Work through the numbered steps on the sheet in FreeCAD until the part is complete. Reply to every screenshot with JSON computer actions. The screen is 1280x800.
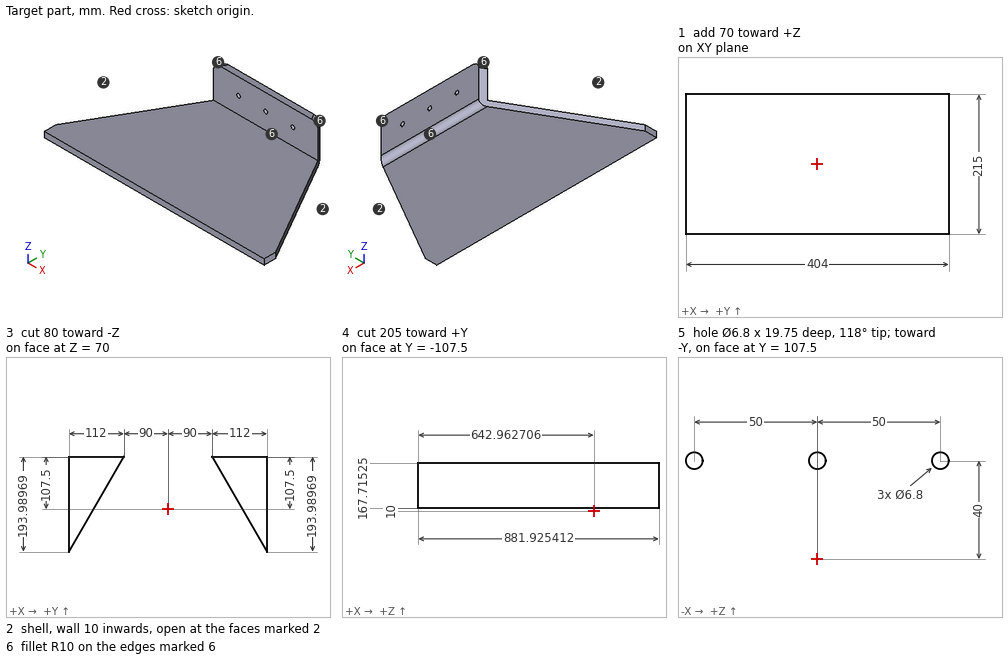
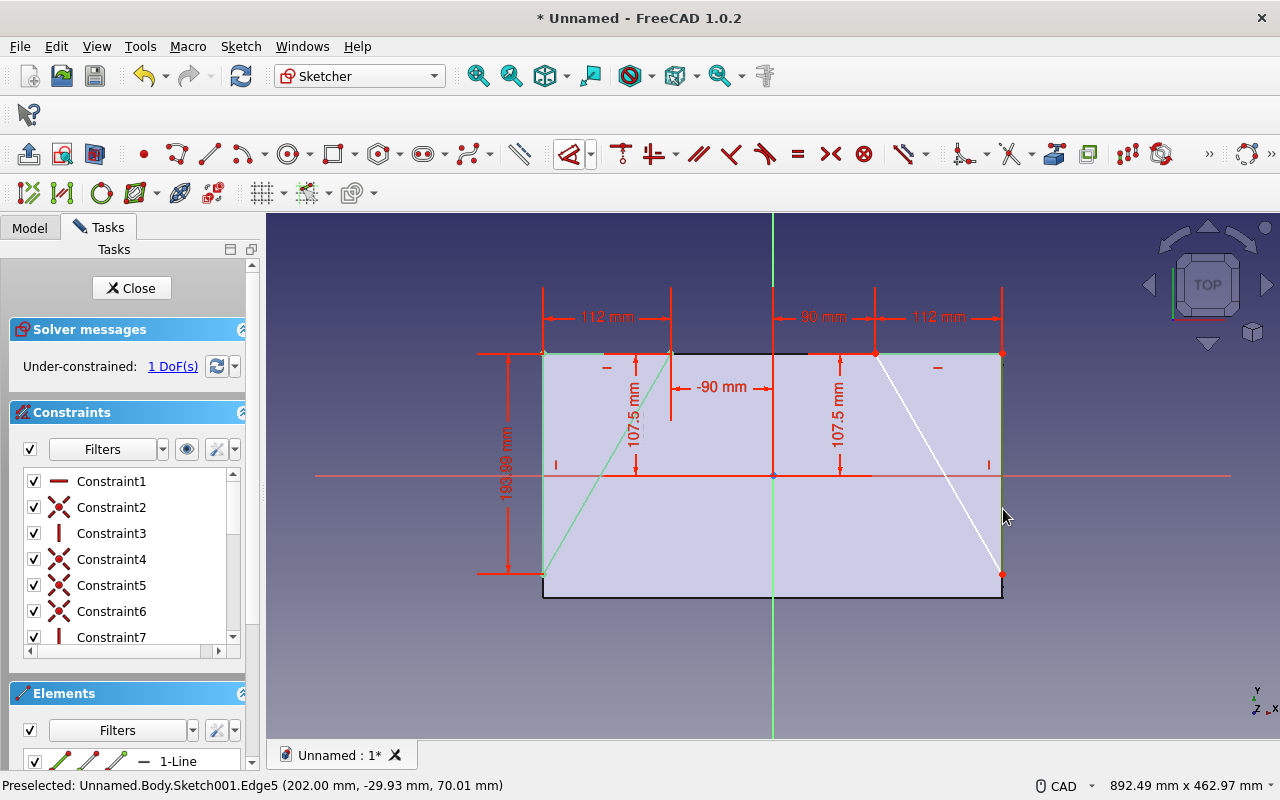
{"action": "left_click", "coordinate": [590, 154]}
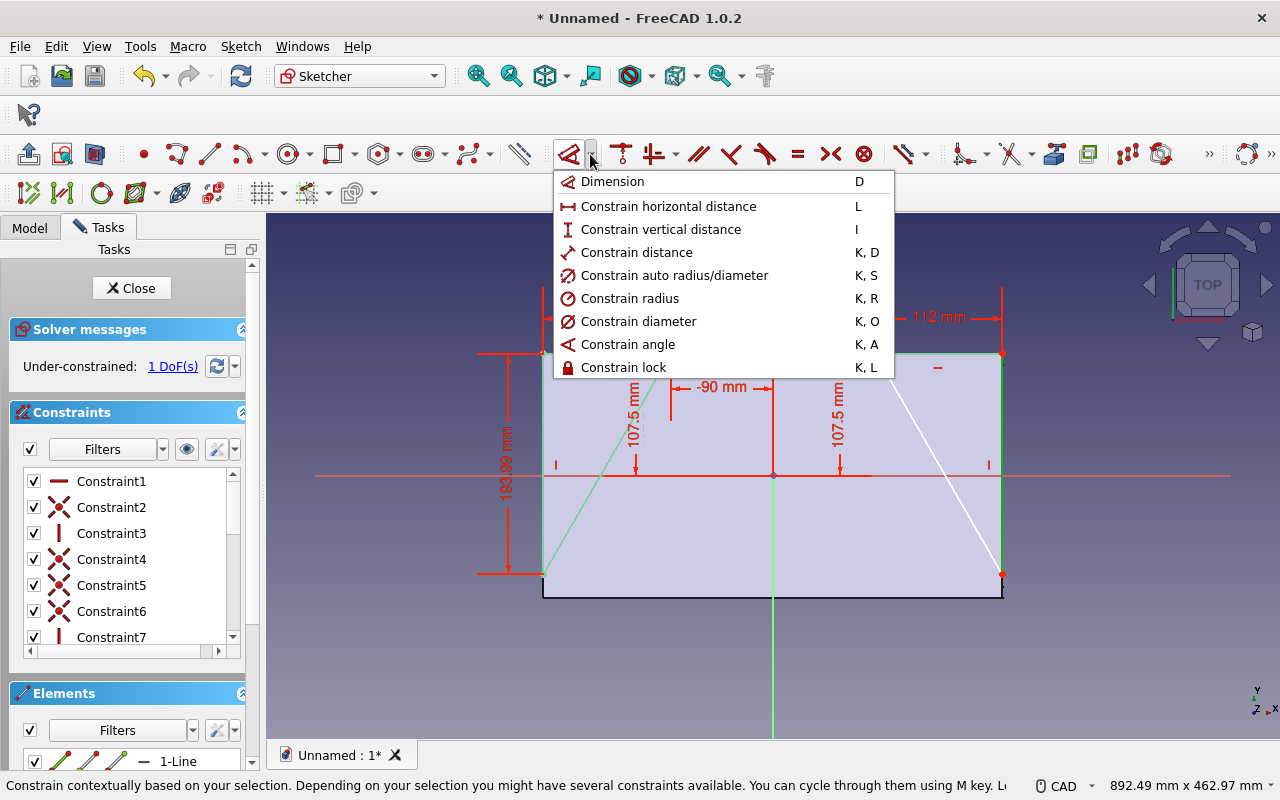
{"action": "left_click", "coordinate": [724, 230]}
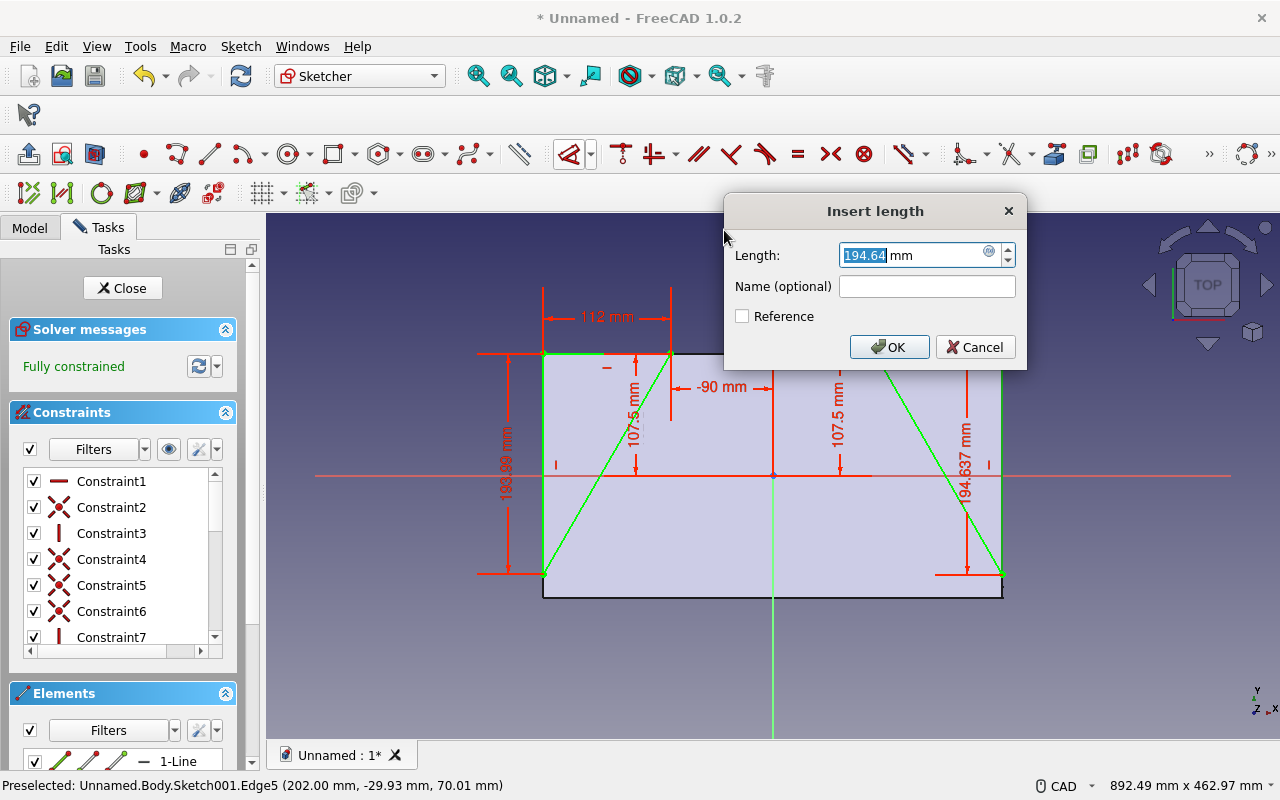
{"action": "type", "text": "193.98969"}
{"action": "key", "text": "Return"}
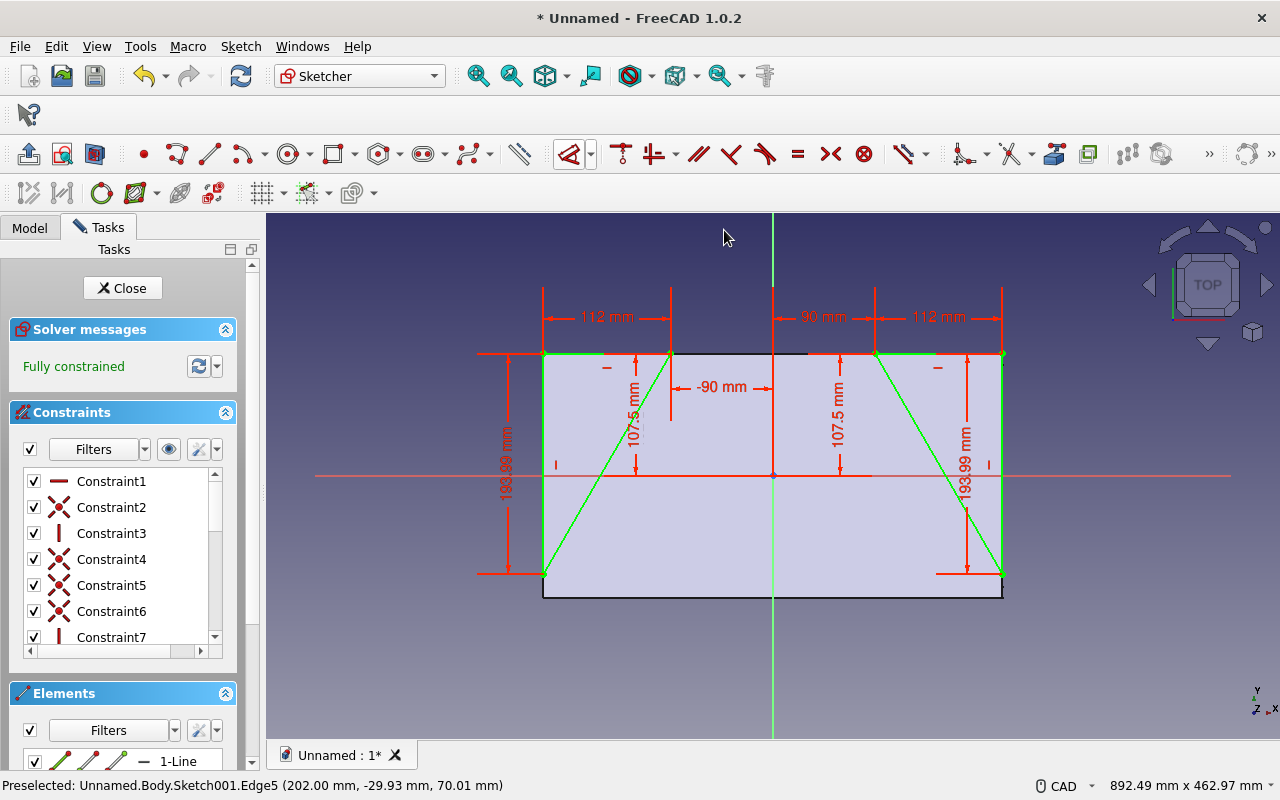
{"action": "left_click", "coordinate": [123, 288]}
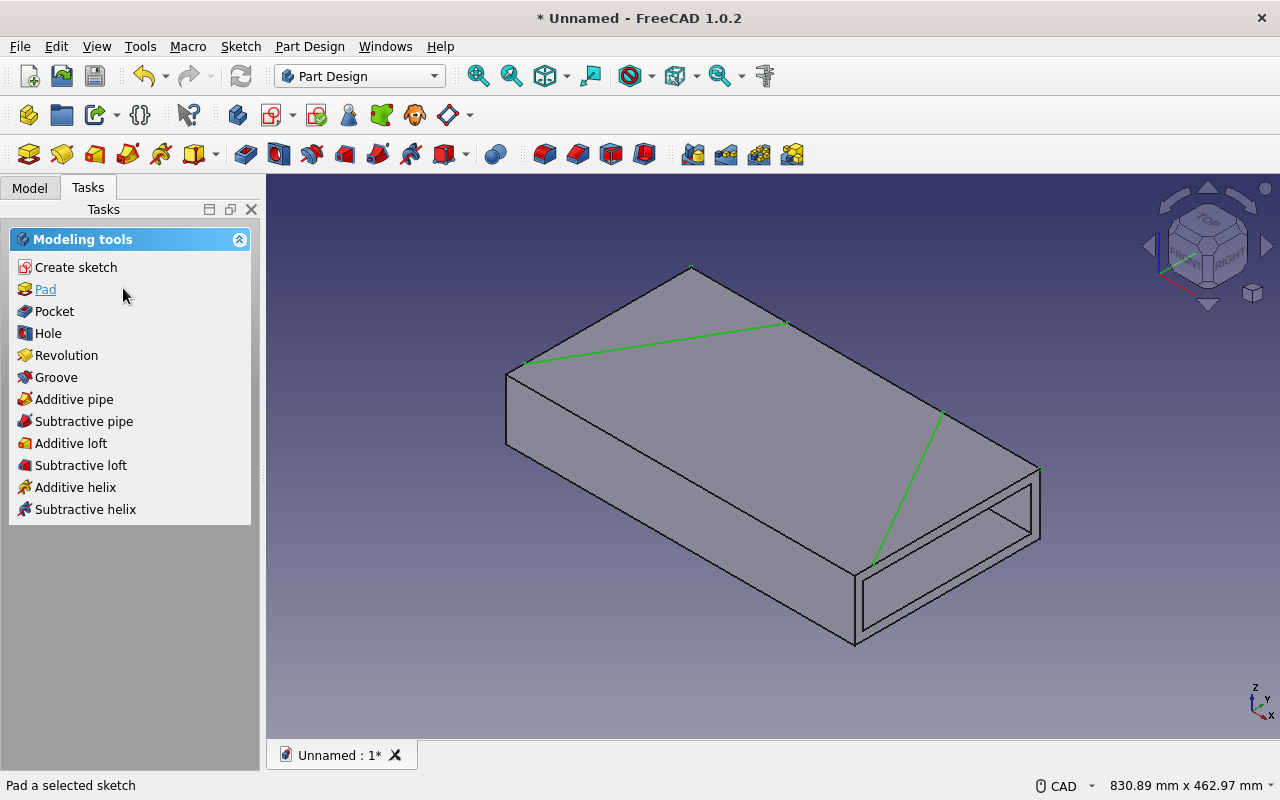
{"action": "left_click", "coordinate": [246, 154]}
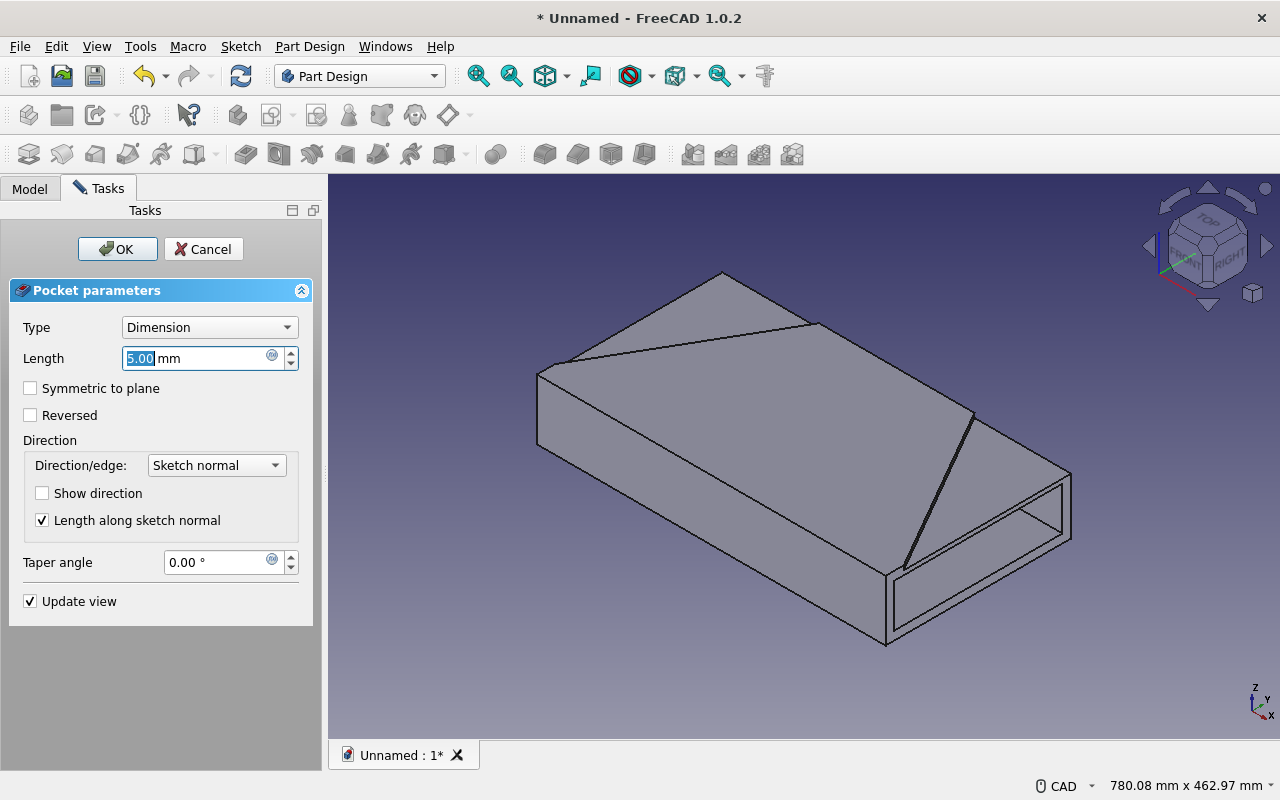
{"action": "type", "text": "80"}
{"action": "key", "text": "Tab"}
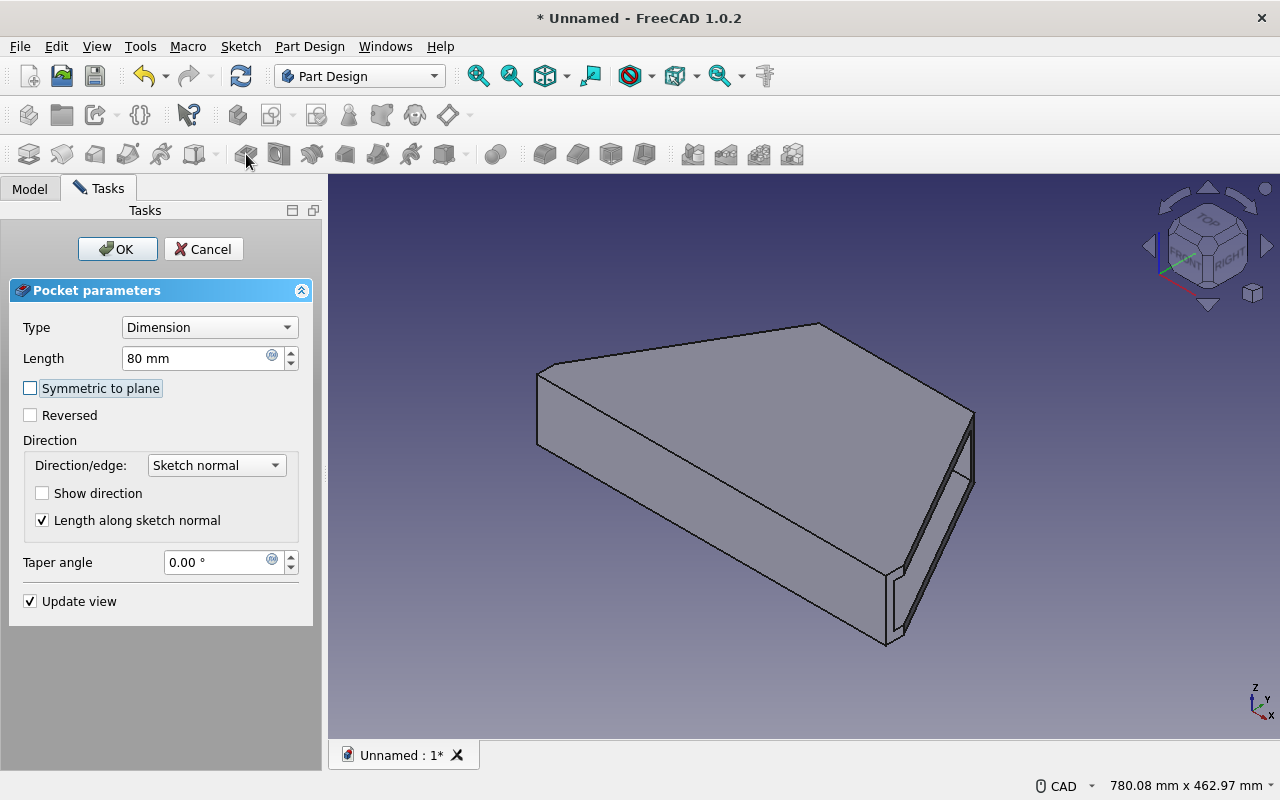
{"action": "left_click", "coordinate": [118, 249]}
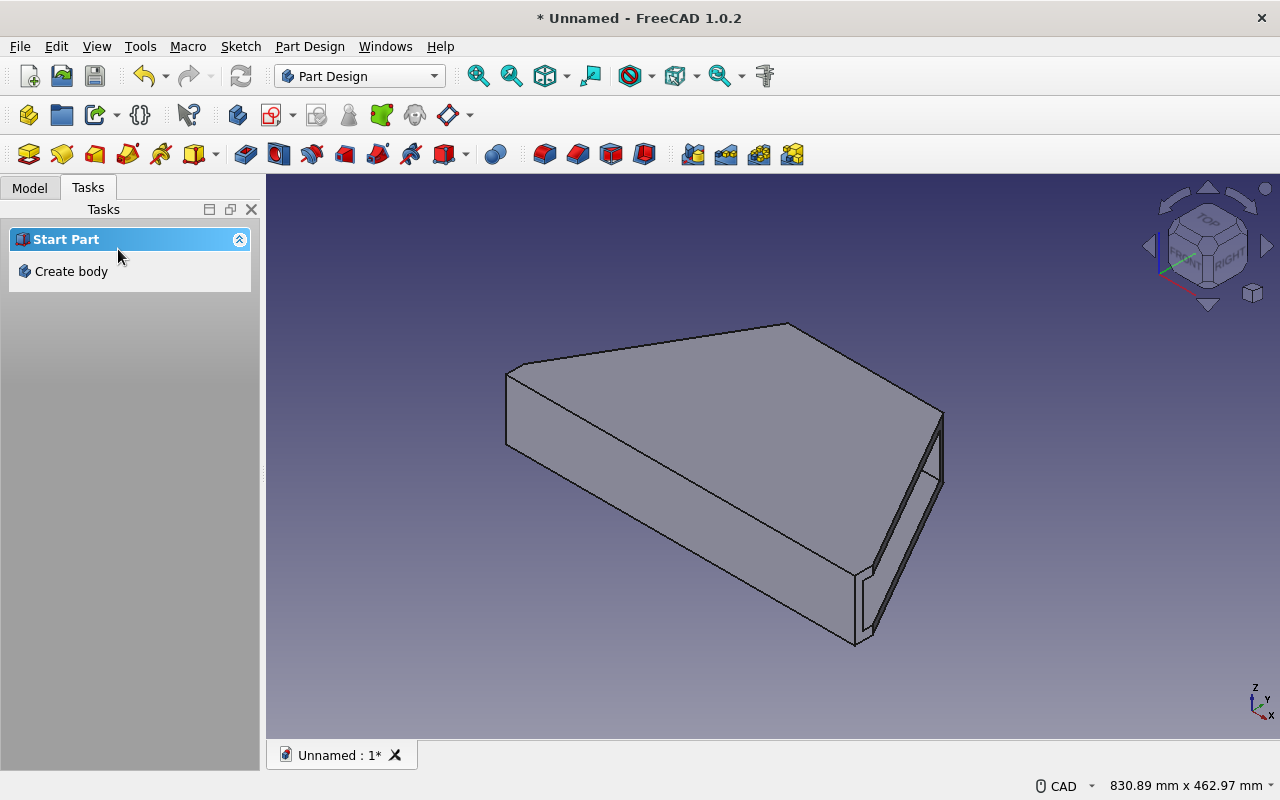
{"action": "left_click", "coordinate": [780, 567]}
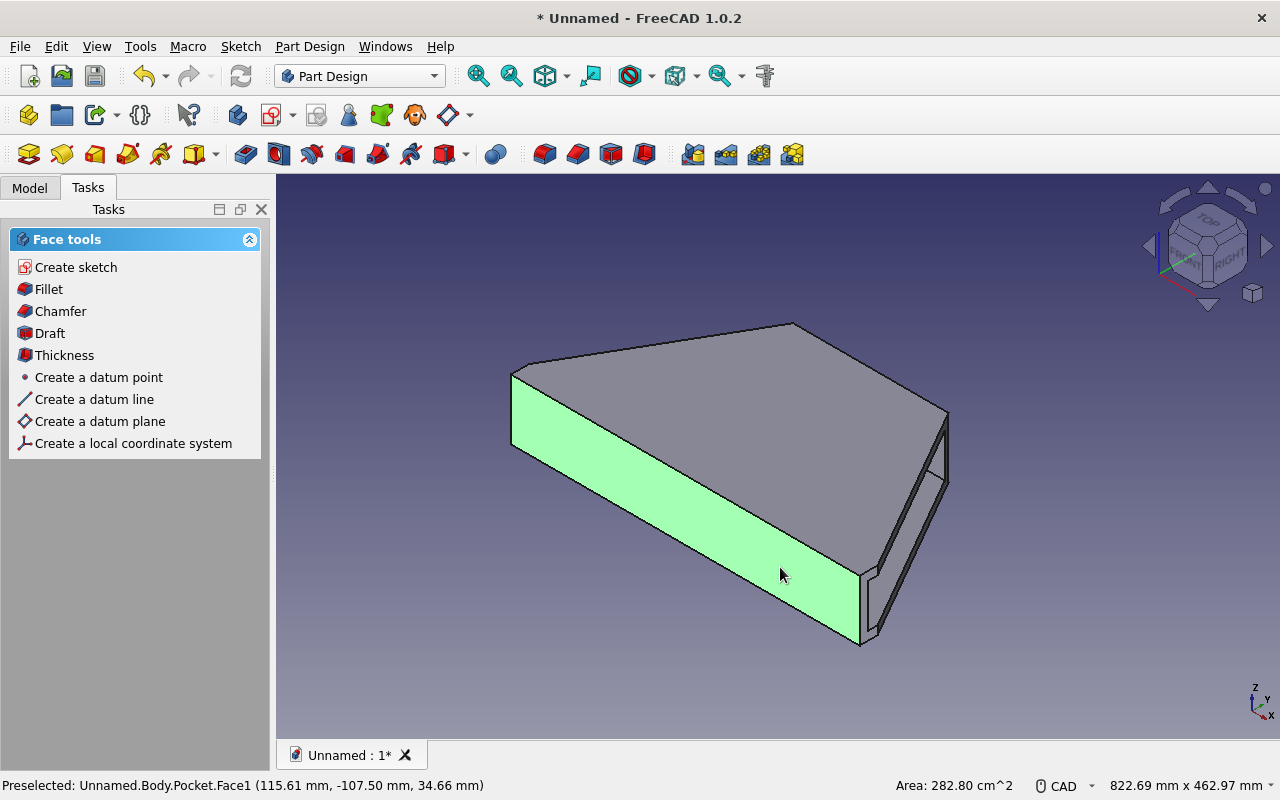
{"action": "left_click", "coordinate": [270, 116]}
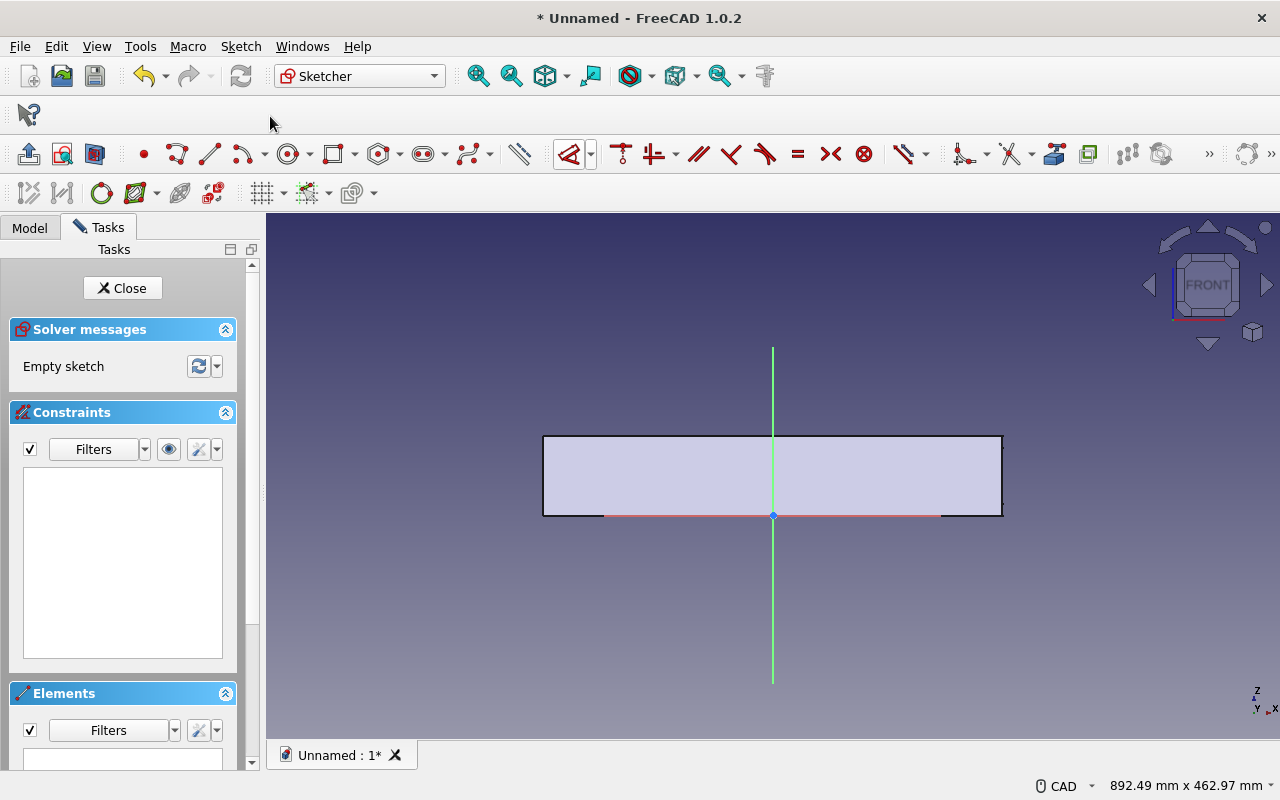
{"action": "scroll", "coordinate": [900, 550], "scroll_direction": "down", "scroll_amount": 3}